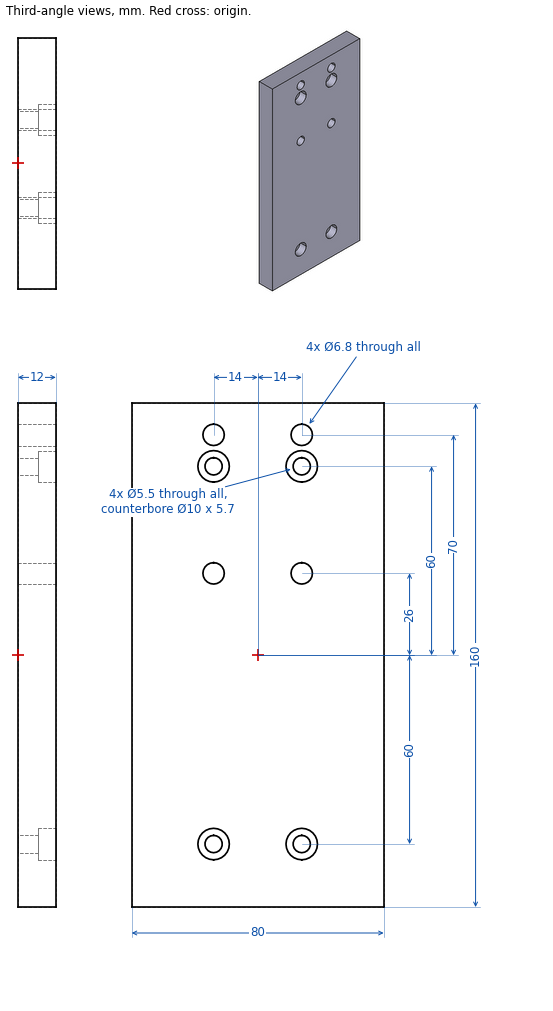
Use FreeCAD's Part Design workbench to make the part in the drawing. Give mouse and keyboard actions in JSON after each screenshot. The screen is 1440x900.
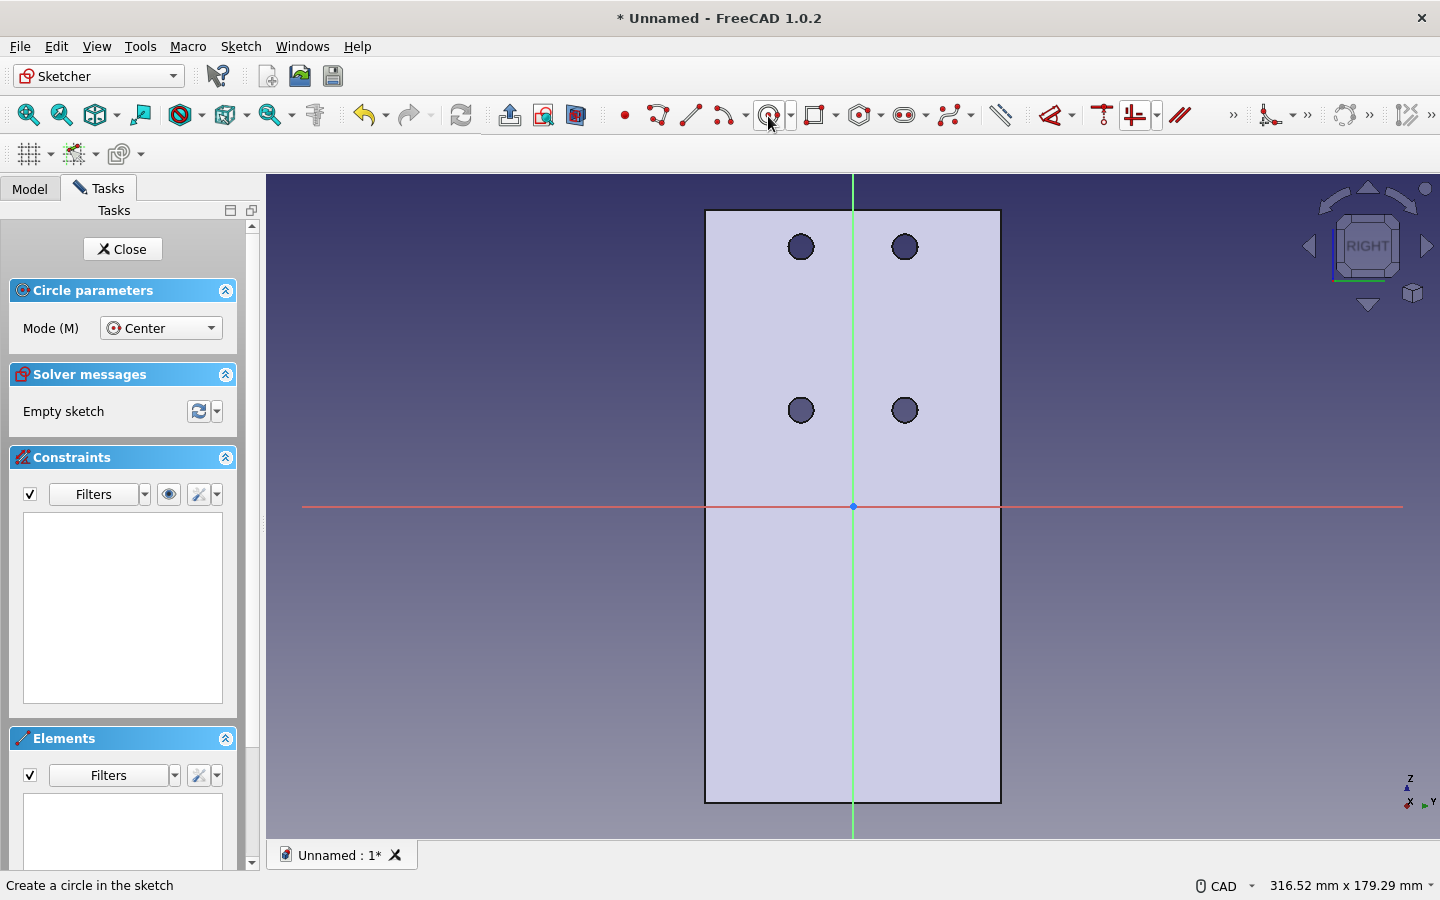
{"action": "scroll", "coordinate": [905, 284], "scroll_direction": "up", "scroll_amount": 4}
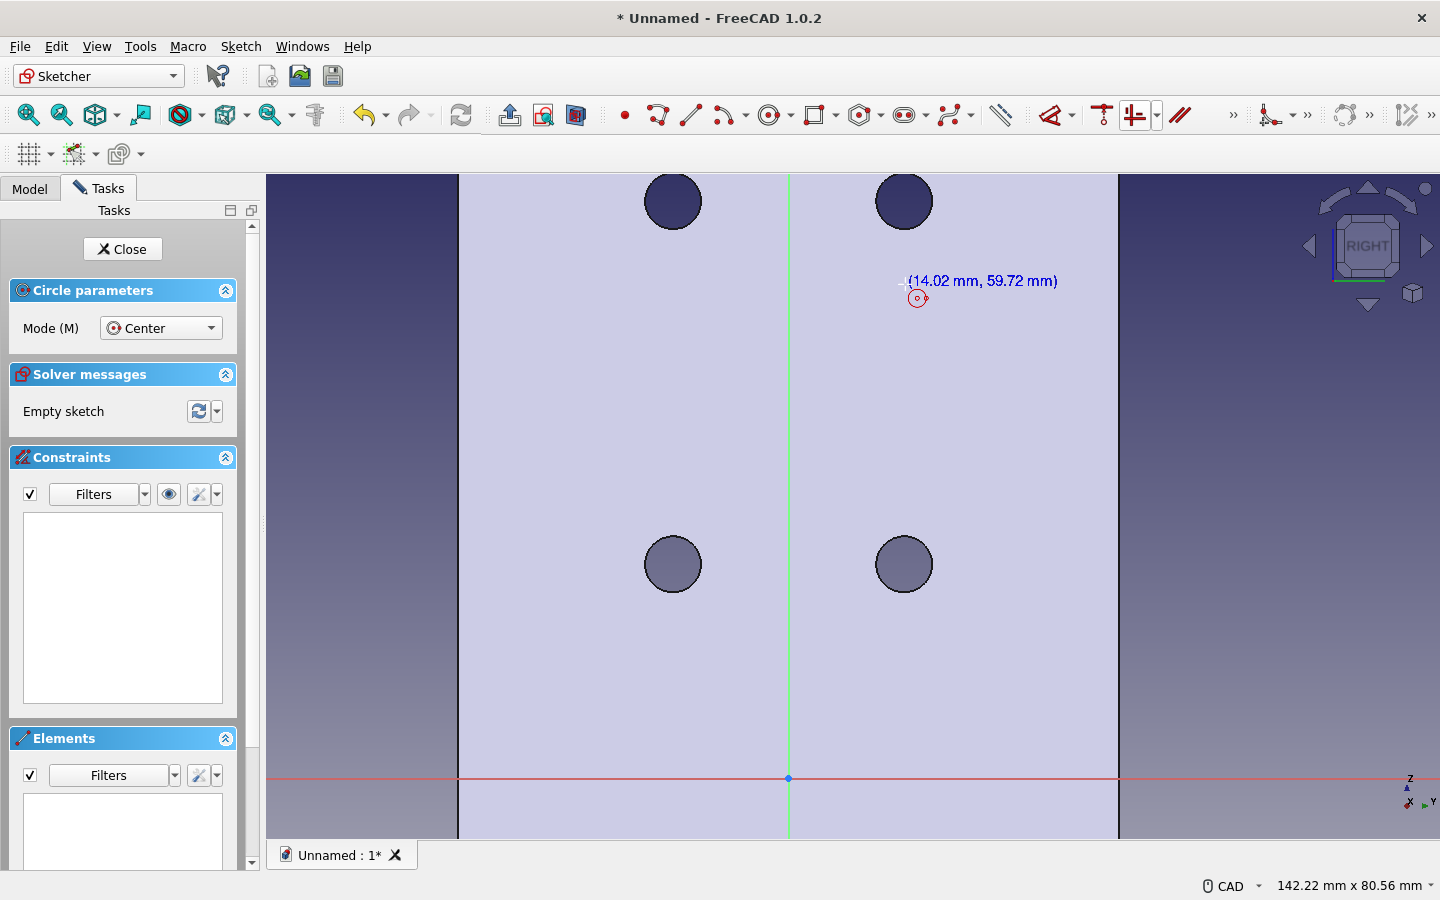
{"action": "left_click", "coordinate": [904, 284]}
{"action": "left_click", "coordinate": [920, 268]}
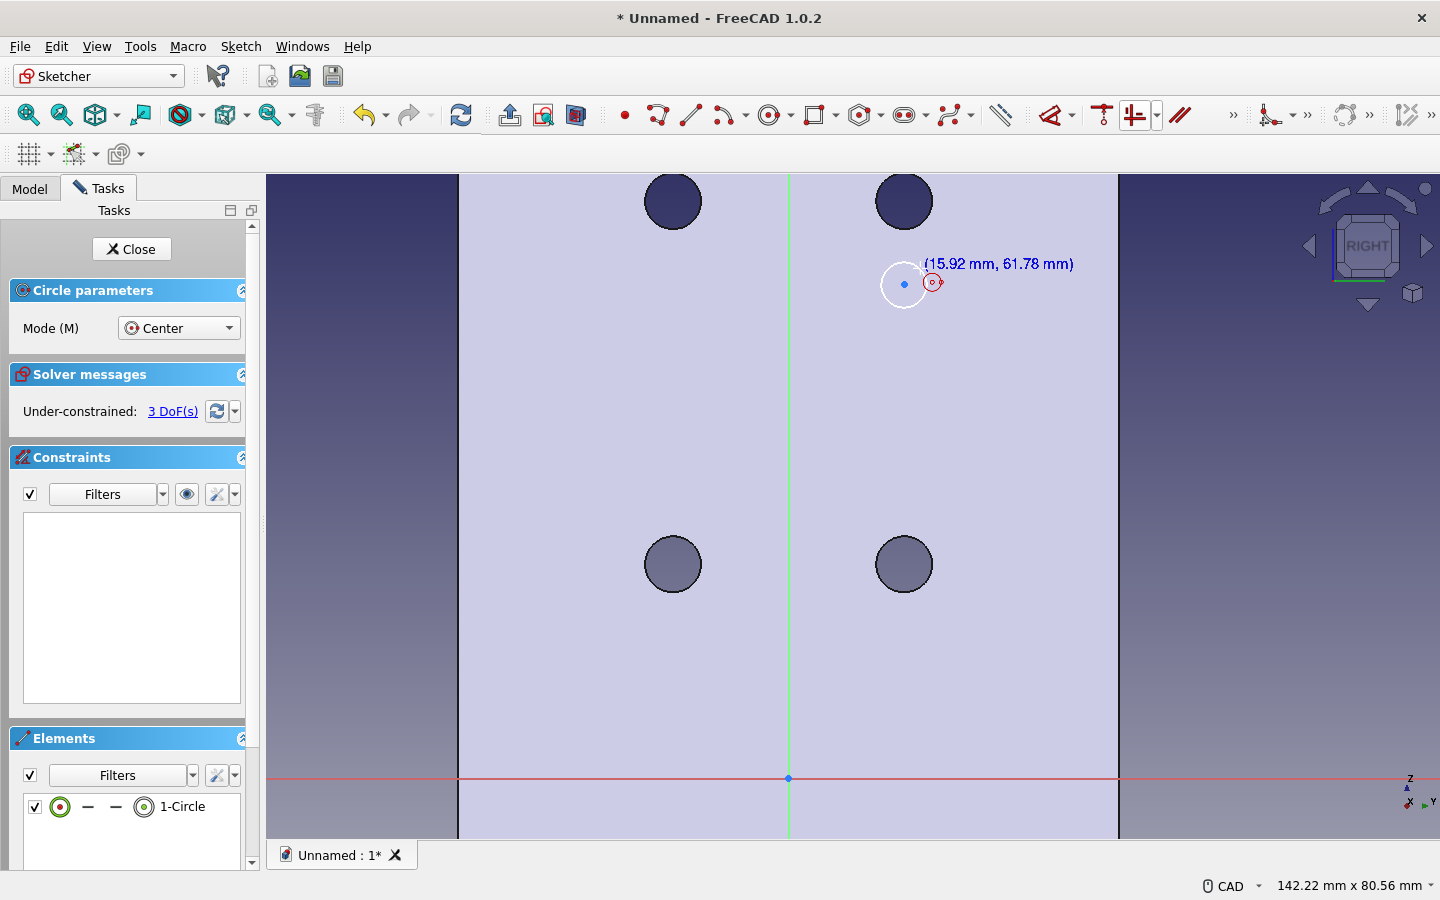
{"action": "left_click", "coordinate": [673, 284]}
{"action": "left_click", "coordinate": [689, 268]}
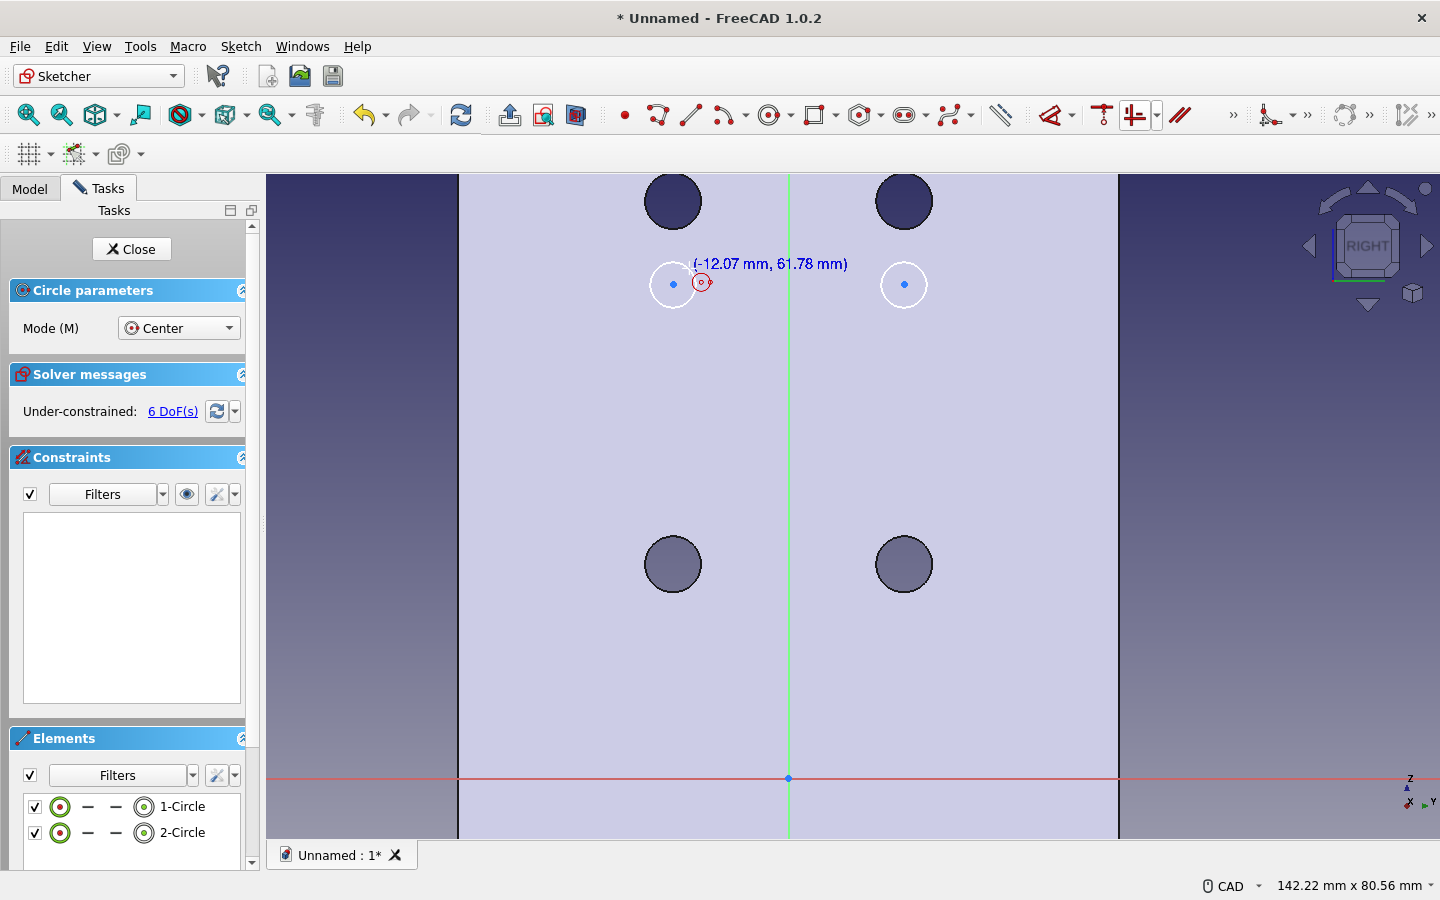
{"action": "scroll", "coordinate": [781, 284], "scroll_direction": "down", "scroll_amount": 4}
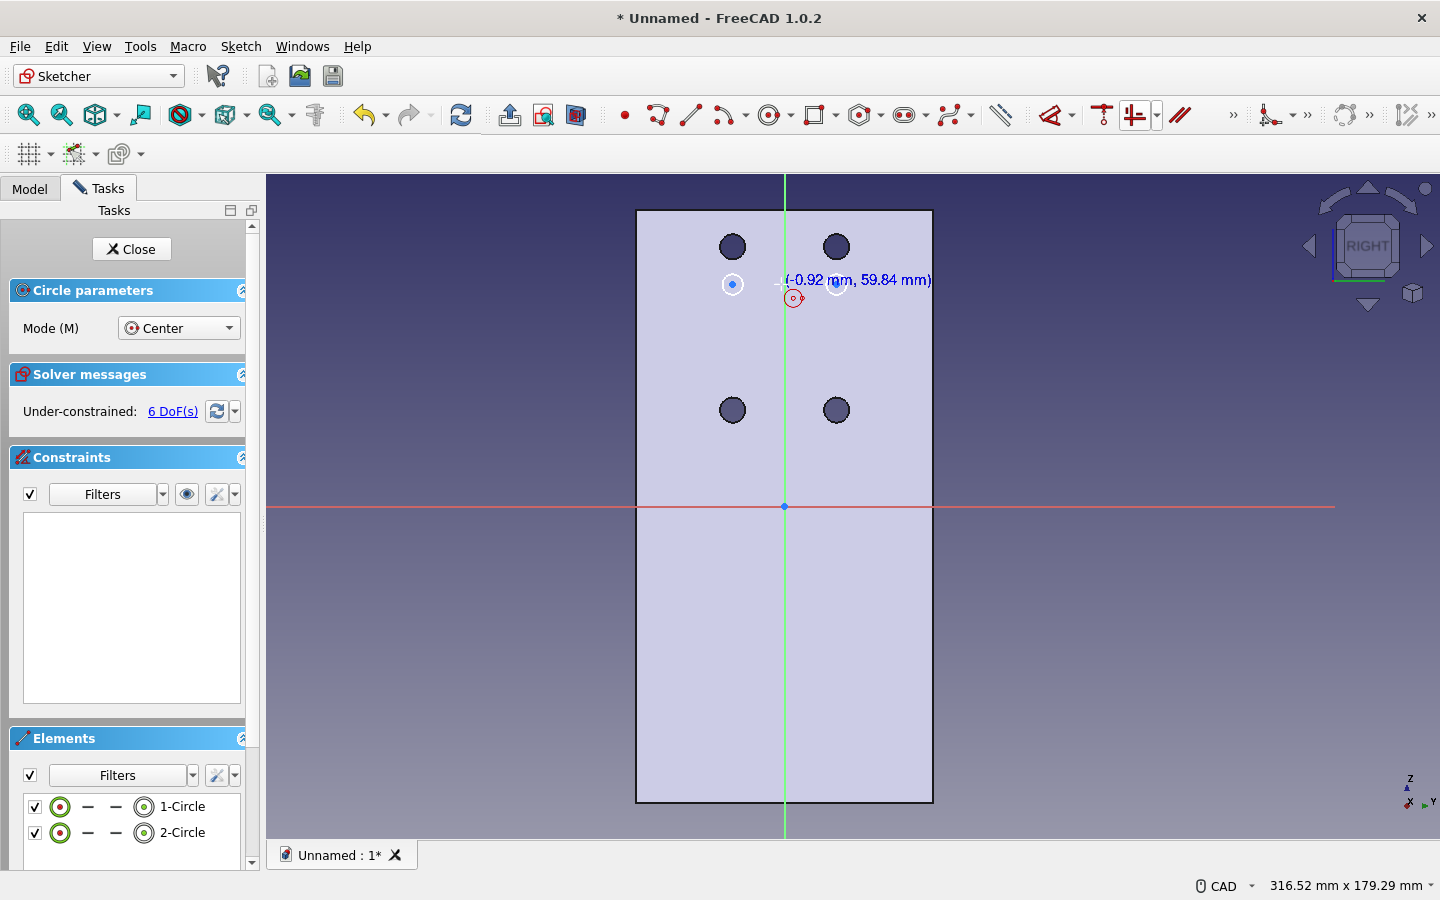
{"action": "scroll", "coordinate": [837, 729], "scroll_direction": "up", "scroll_amount": 4}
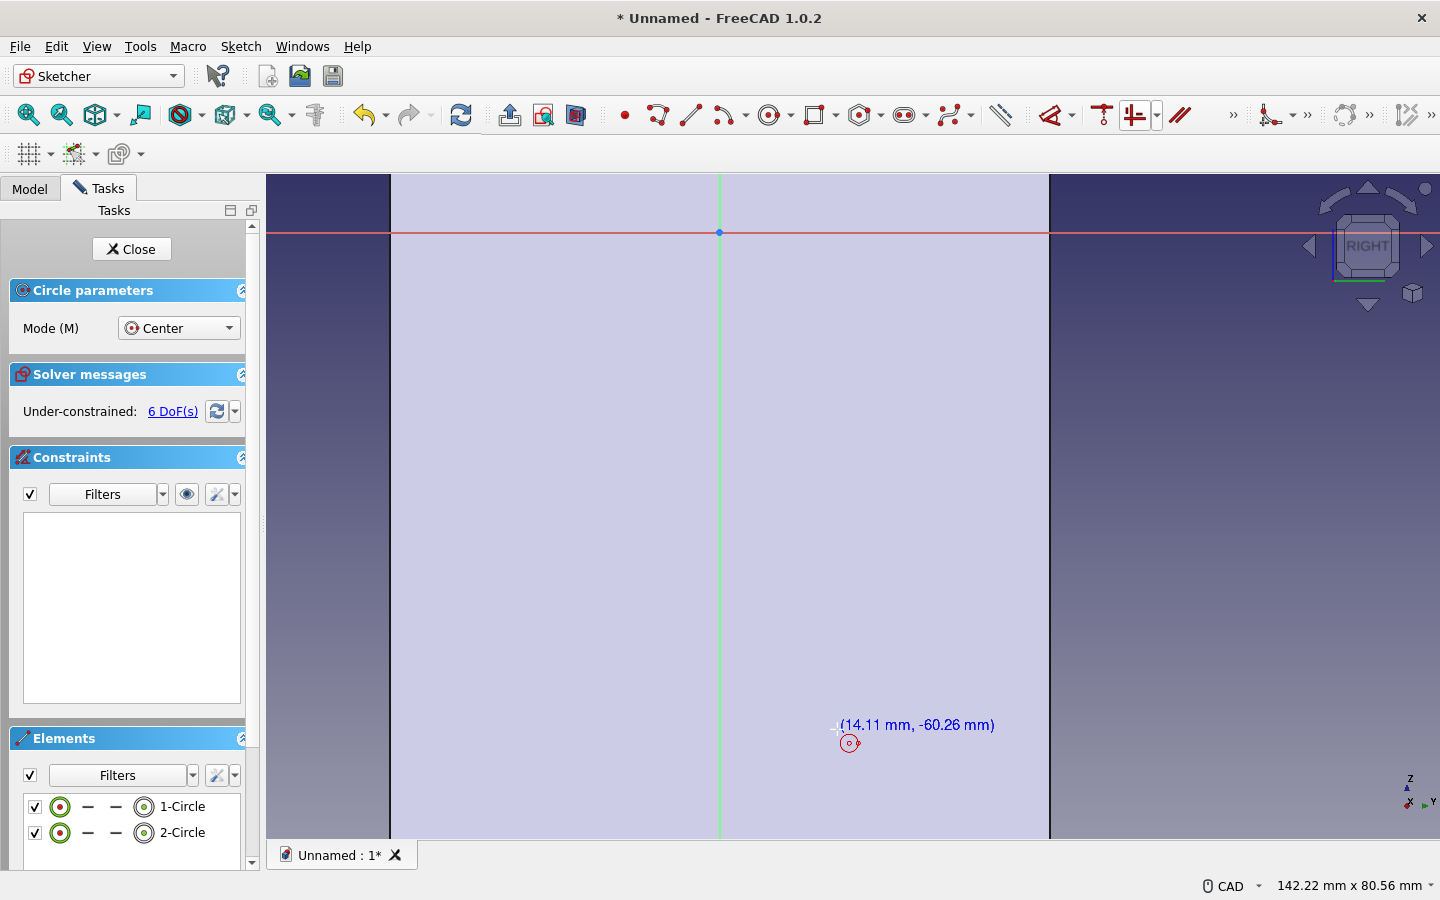
{"action": "left_click", "coordinate": [835, 728]}
{"action": "left_click", "coordinate": [852, 712]}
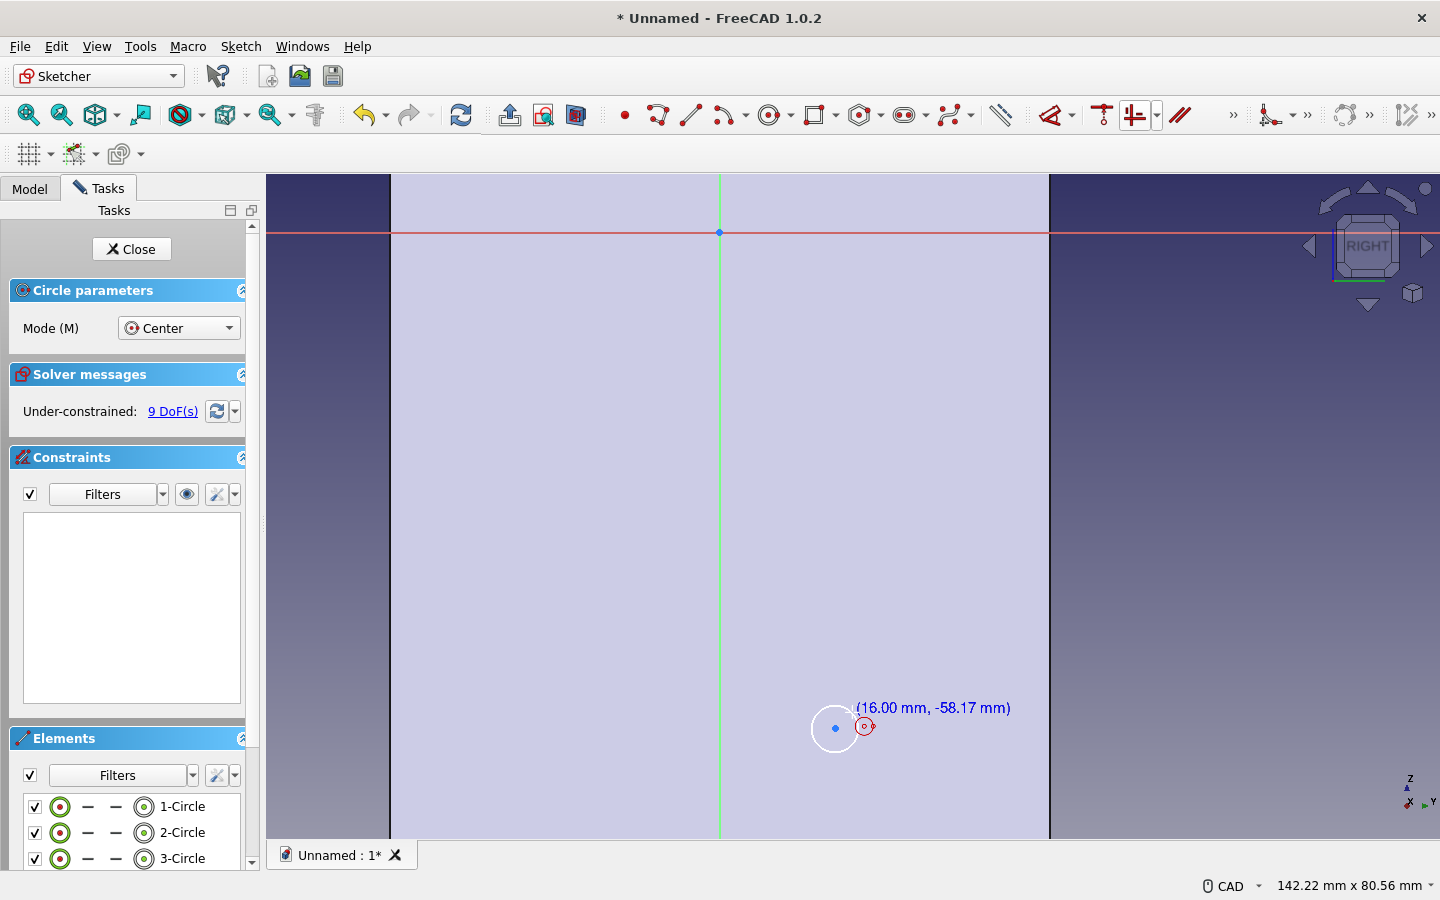
{"action": "left_click", "coordinate": [604, 728]}
{"action": "left_click", "coordinate": [620, 712]}
{"action": "key", "text": "Escape"}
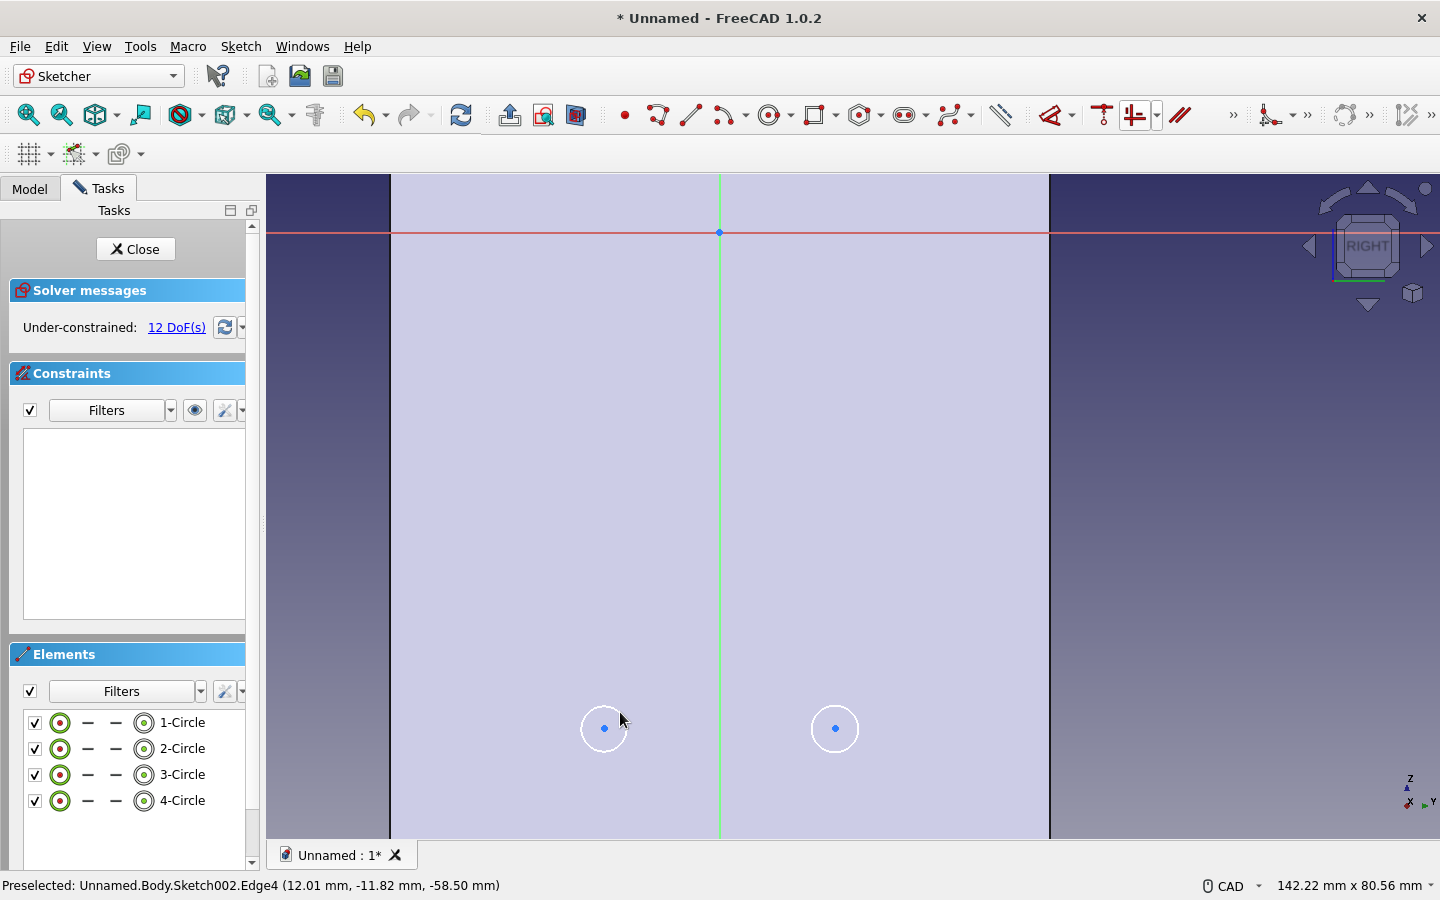
{"action": "scroll", "coordinate": [837, 730], "scroll_direction": "down", "scroll_amount": 4}